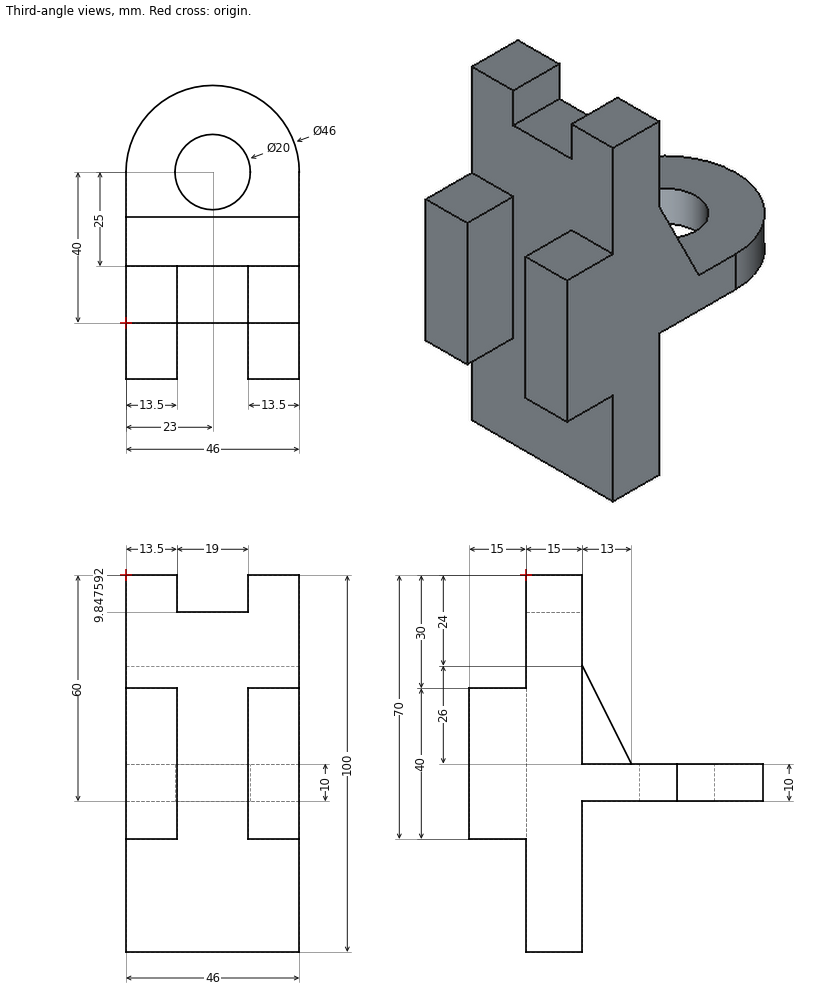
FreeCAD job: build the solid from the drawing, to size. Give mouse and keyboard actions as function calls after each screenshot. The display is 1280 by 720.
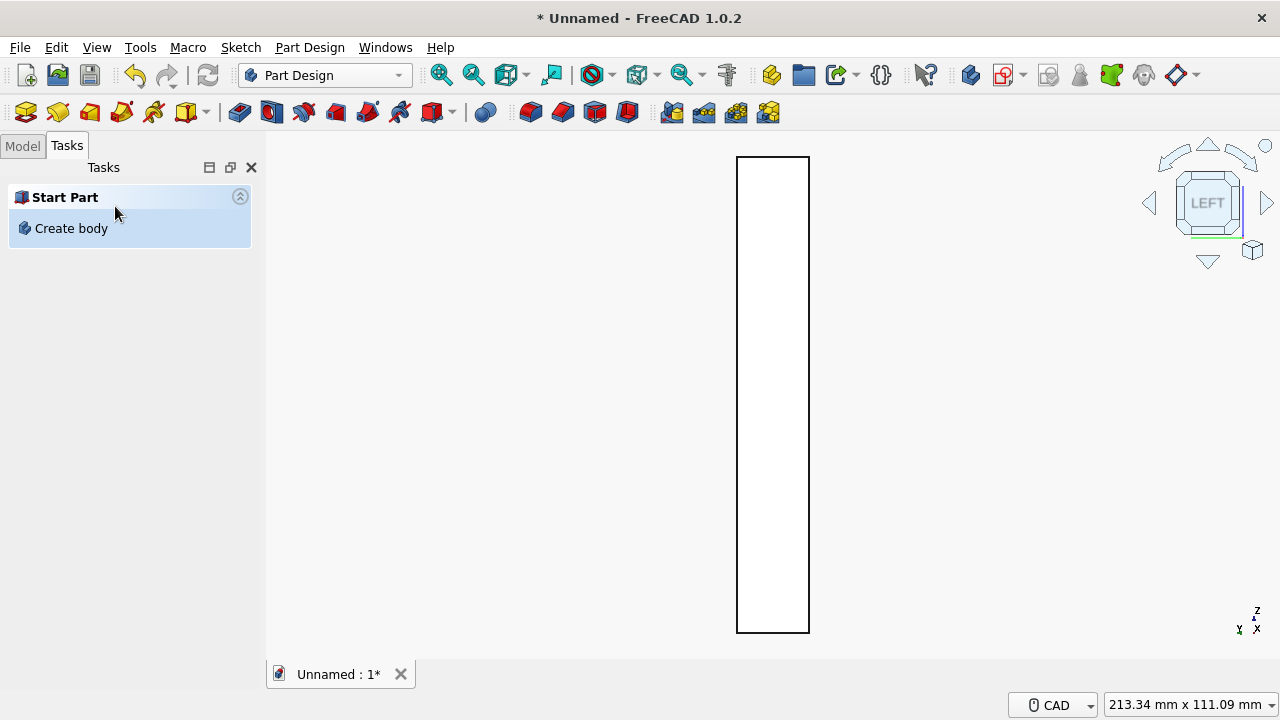
click(773, 258)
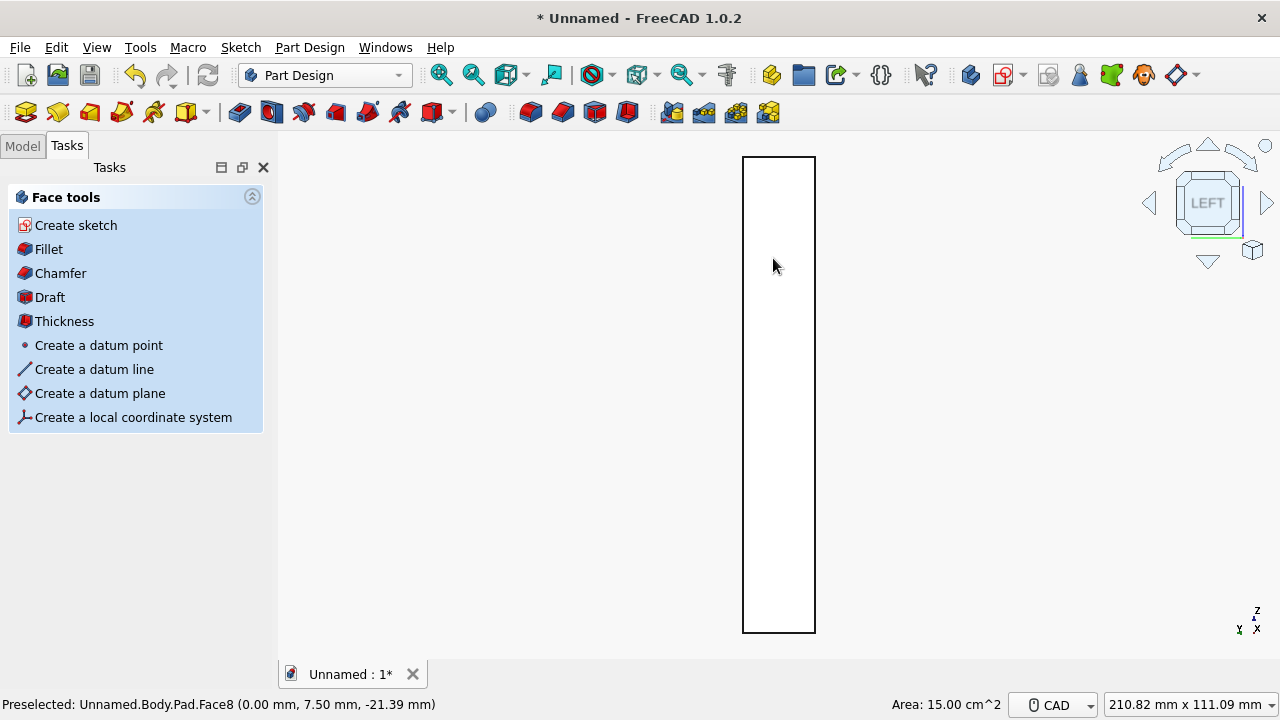
click(1004, 76)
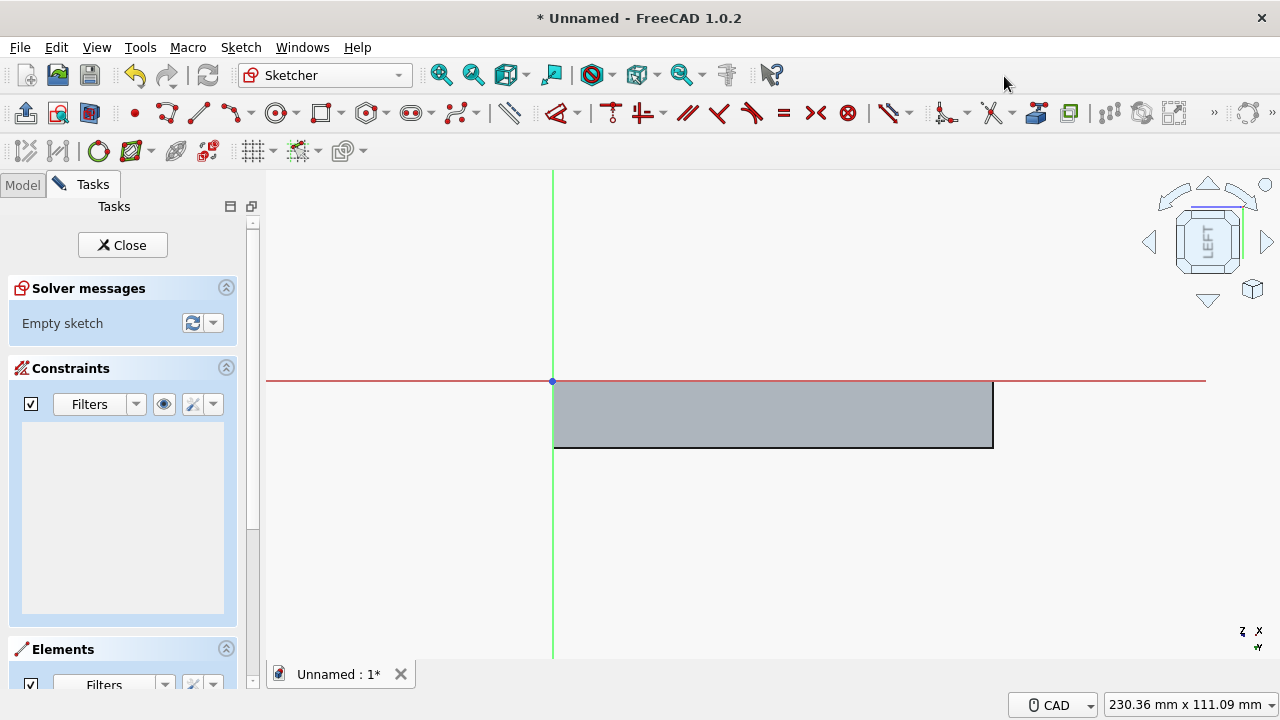
scroll(710, 268, up, 3)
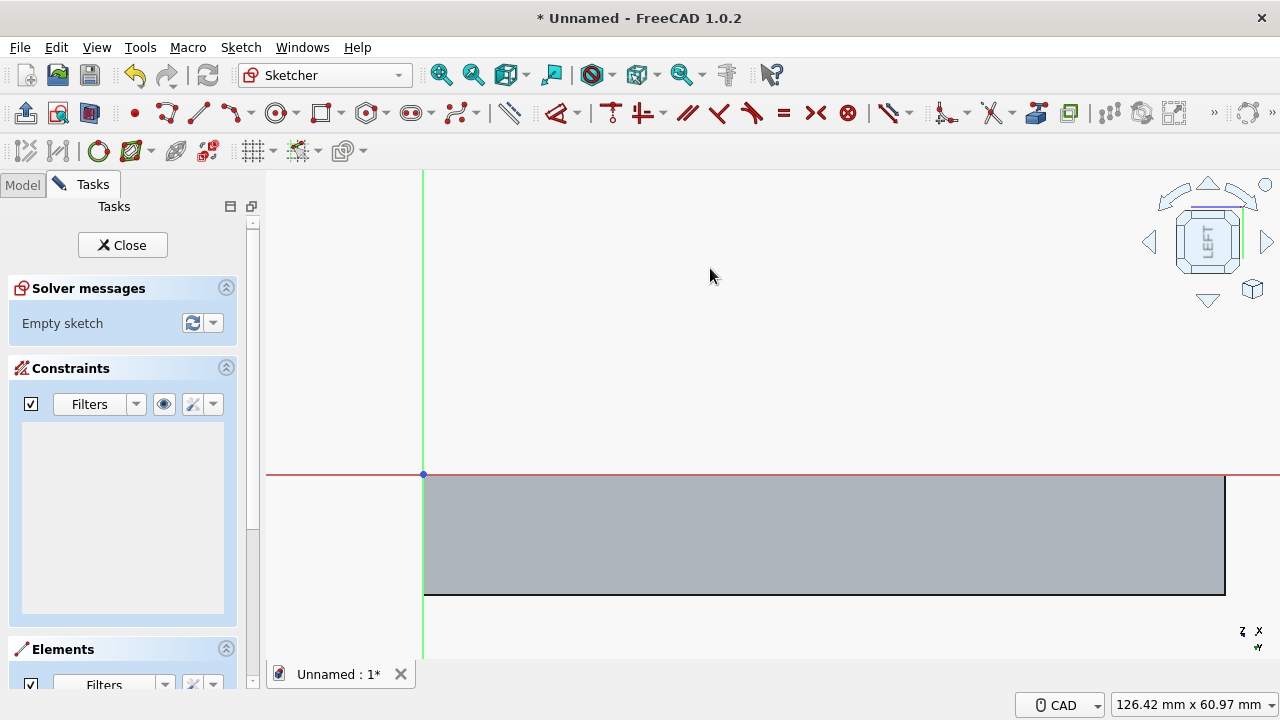
key(g)
key(r)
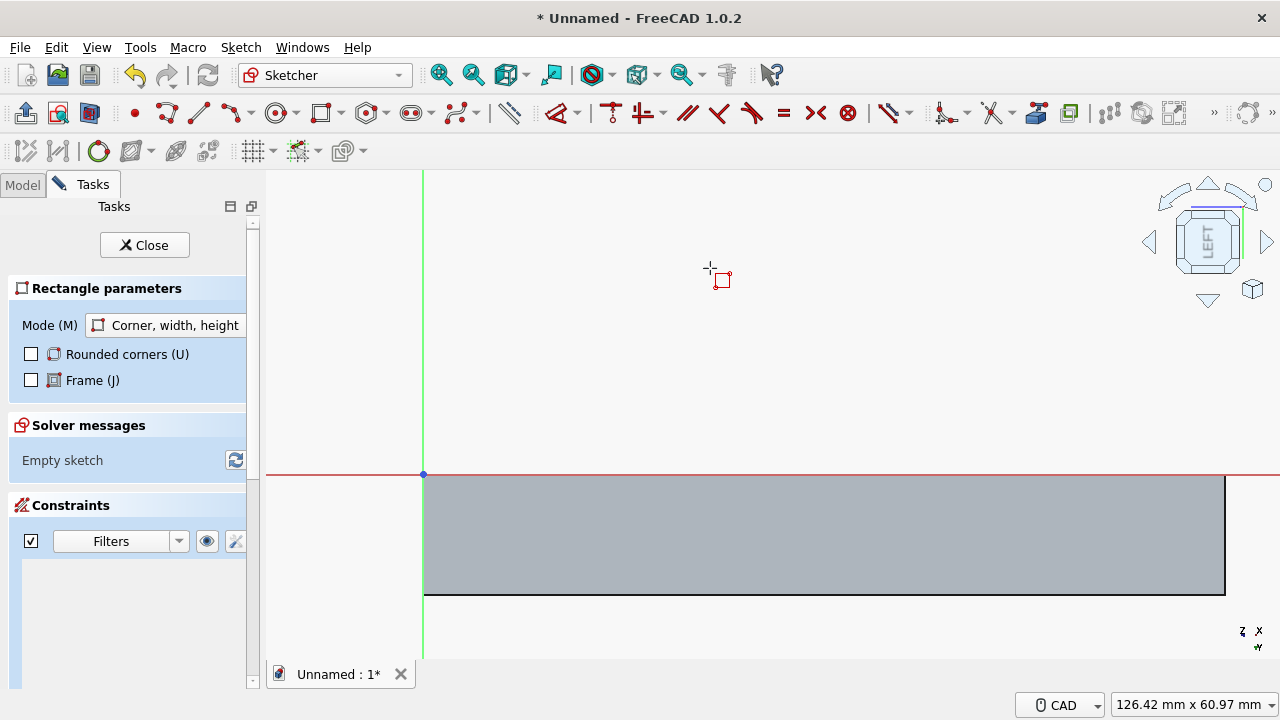
click(664, 354)
click(985, 475)
key(Escape)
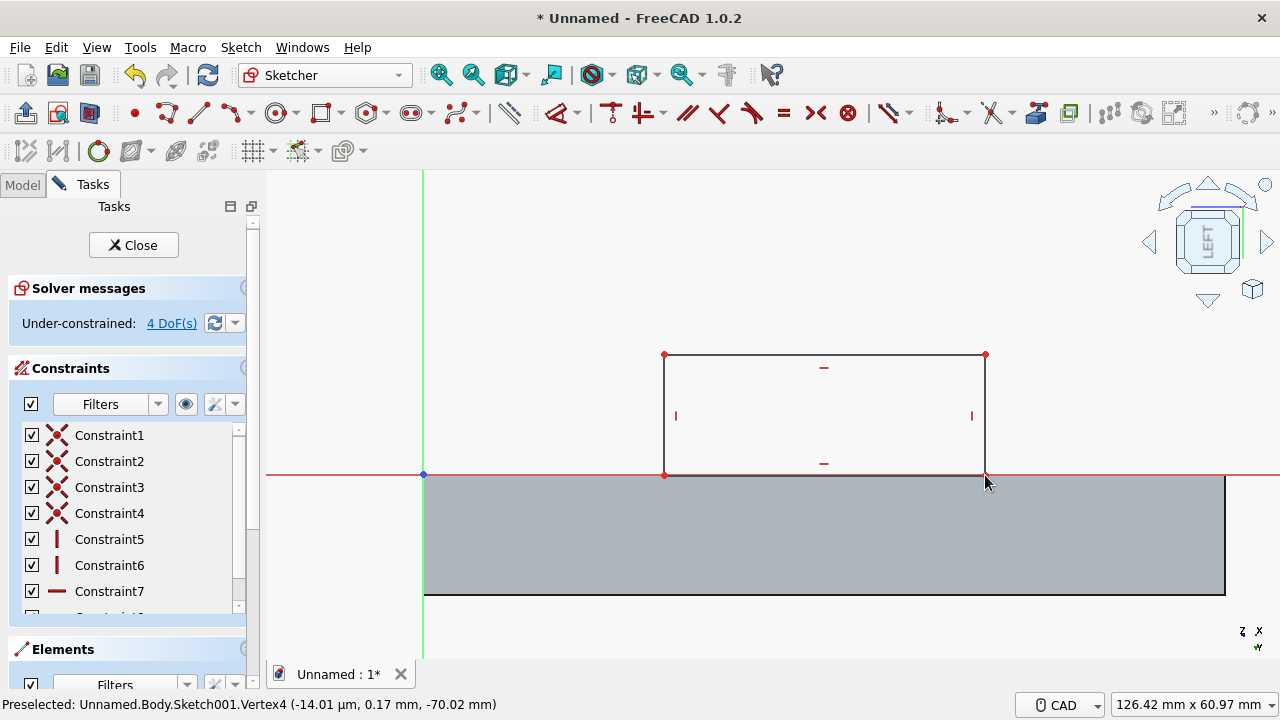
click(664, 476)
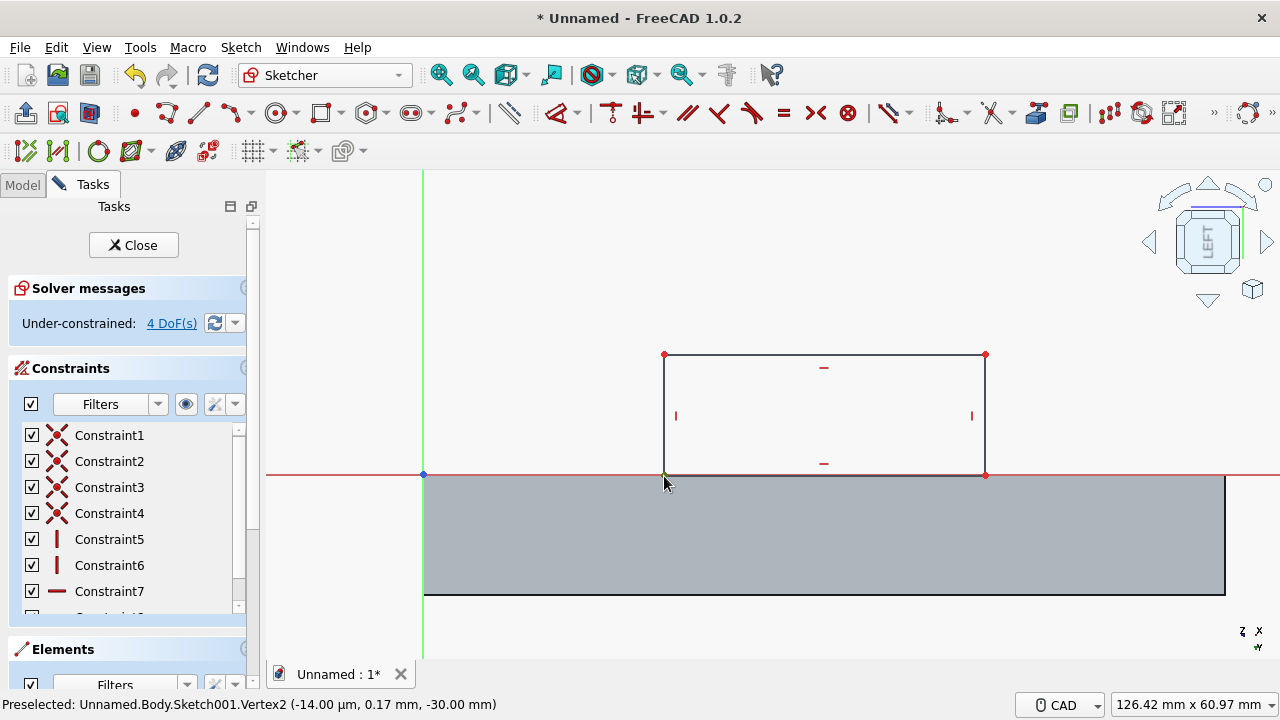
click(353, 475)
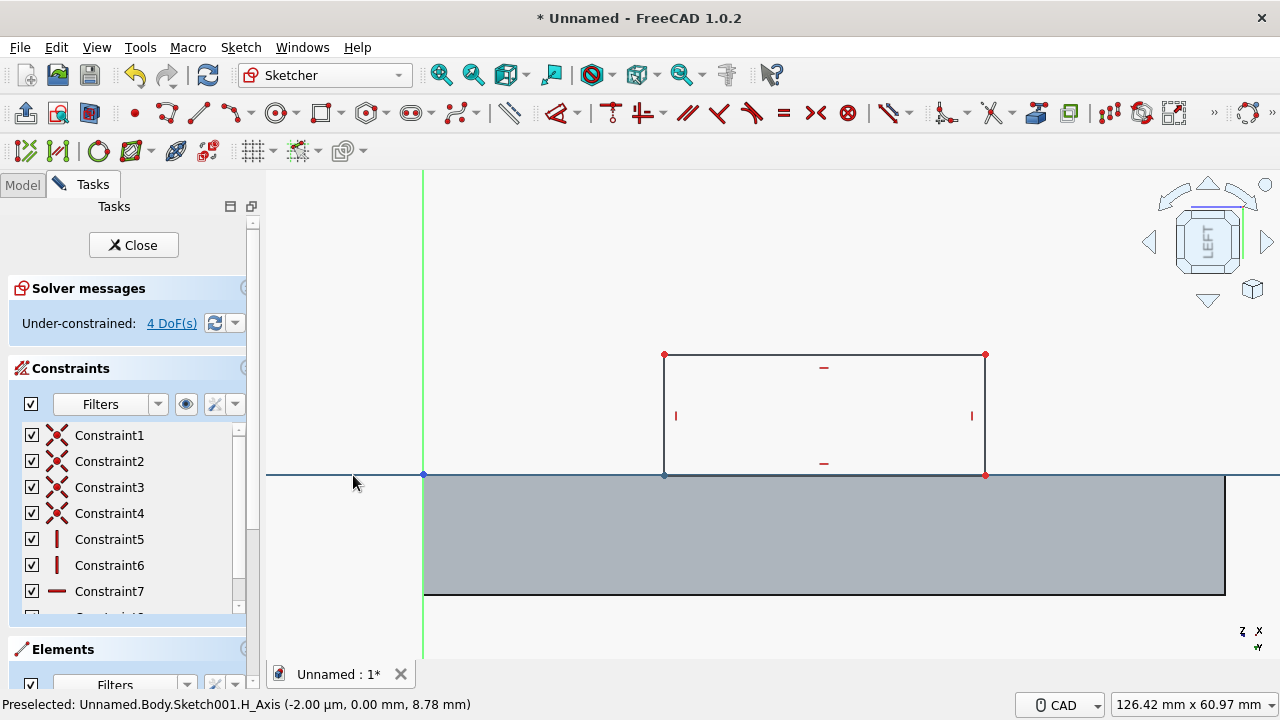
key(c)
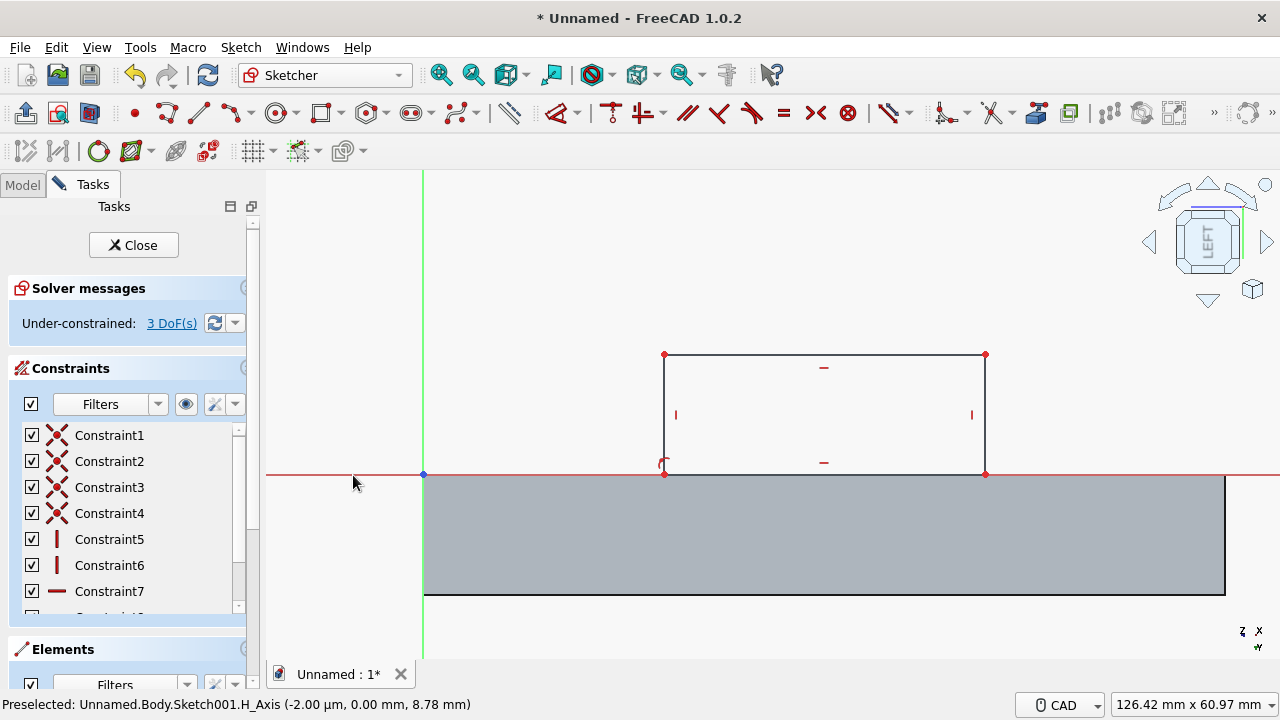
key(d)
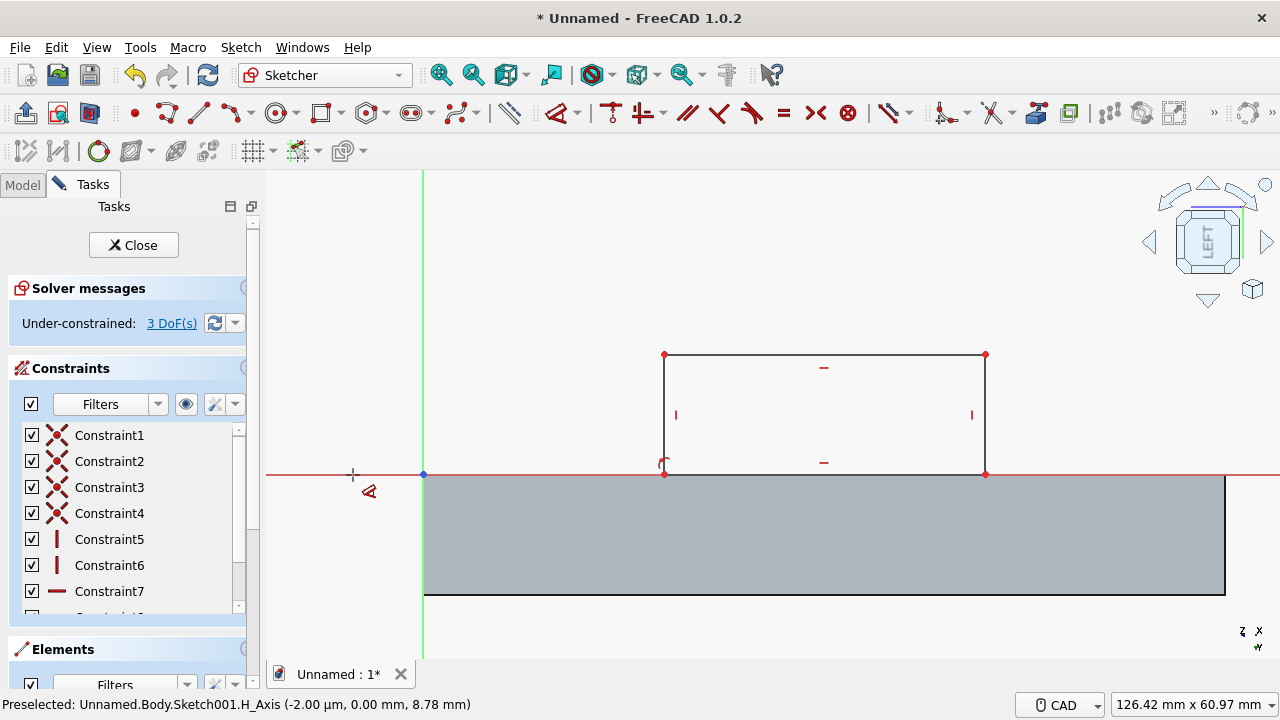
click(664, 391)
click(630, 415)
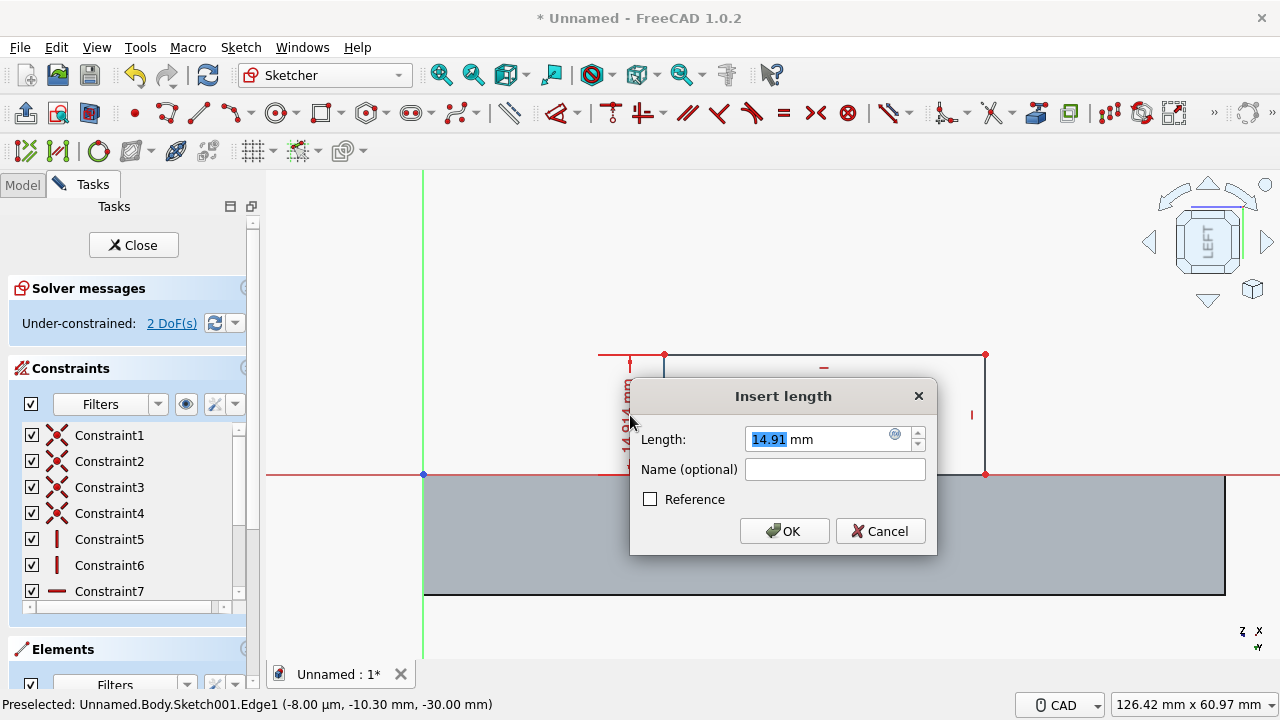
text(15)
key(Return)